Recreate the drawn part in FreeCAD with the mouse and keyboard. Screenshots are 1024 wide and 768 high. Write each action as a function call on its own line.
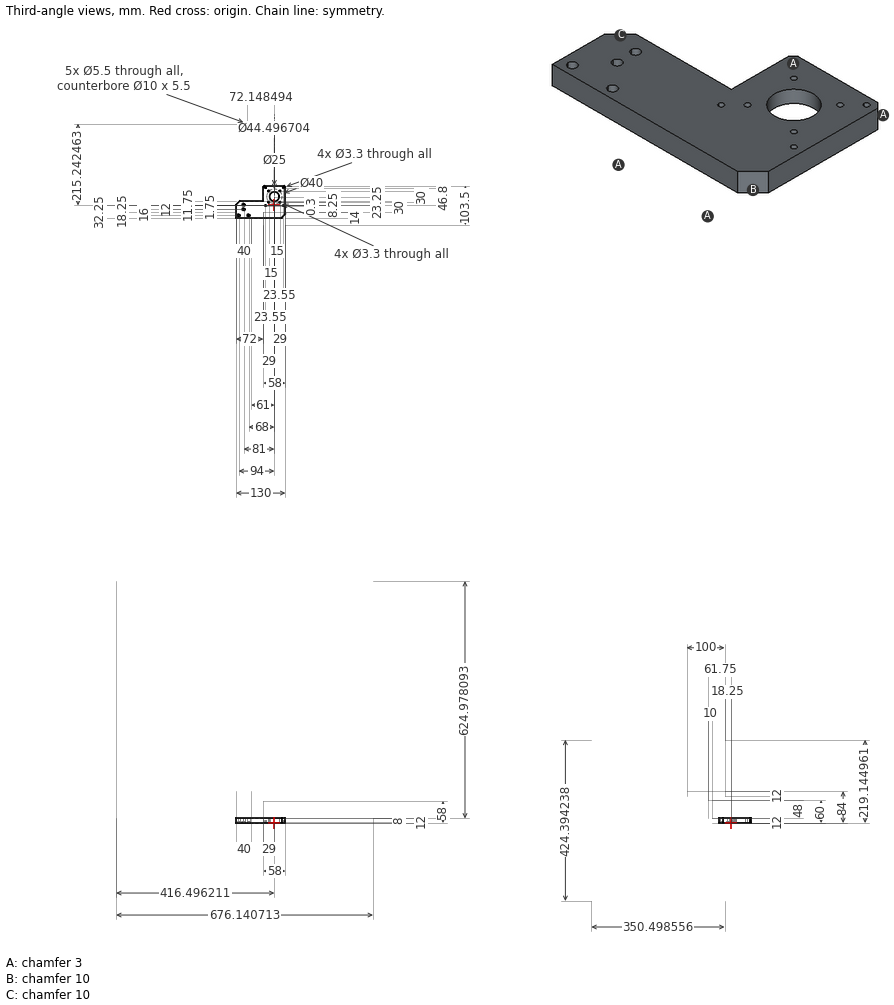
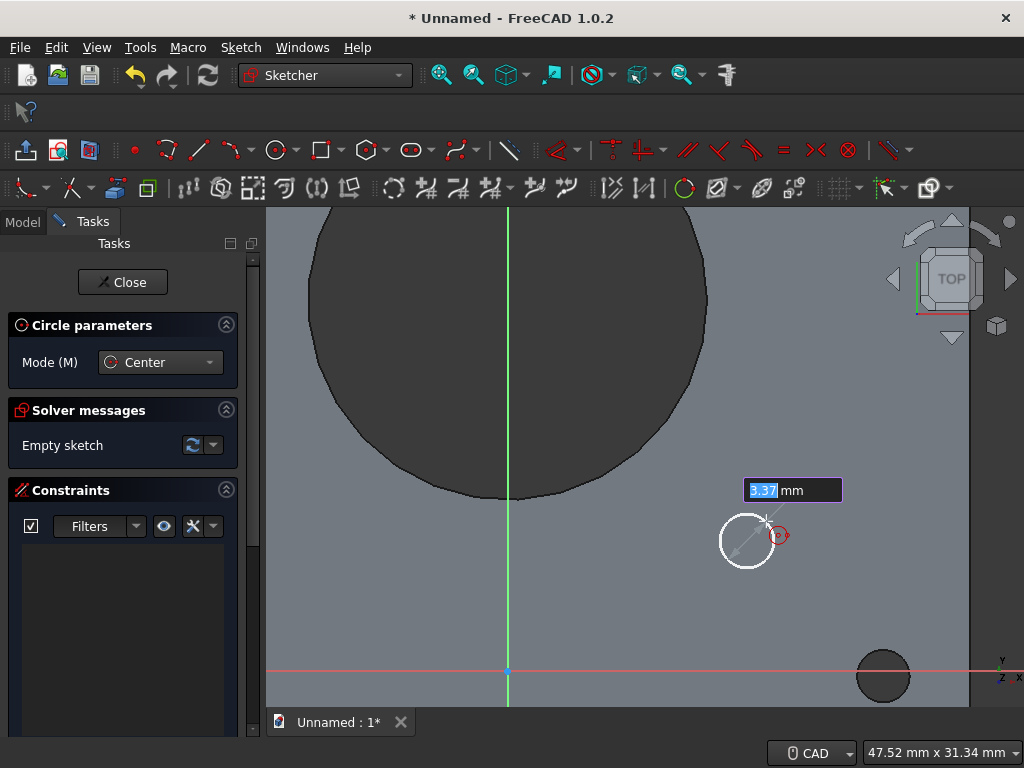
text(3.3)
key(Return)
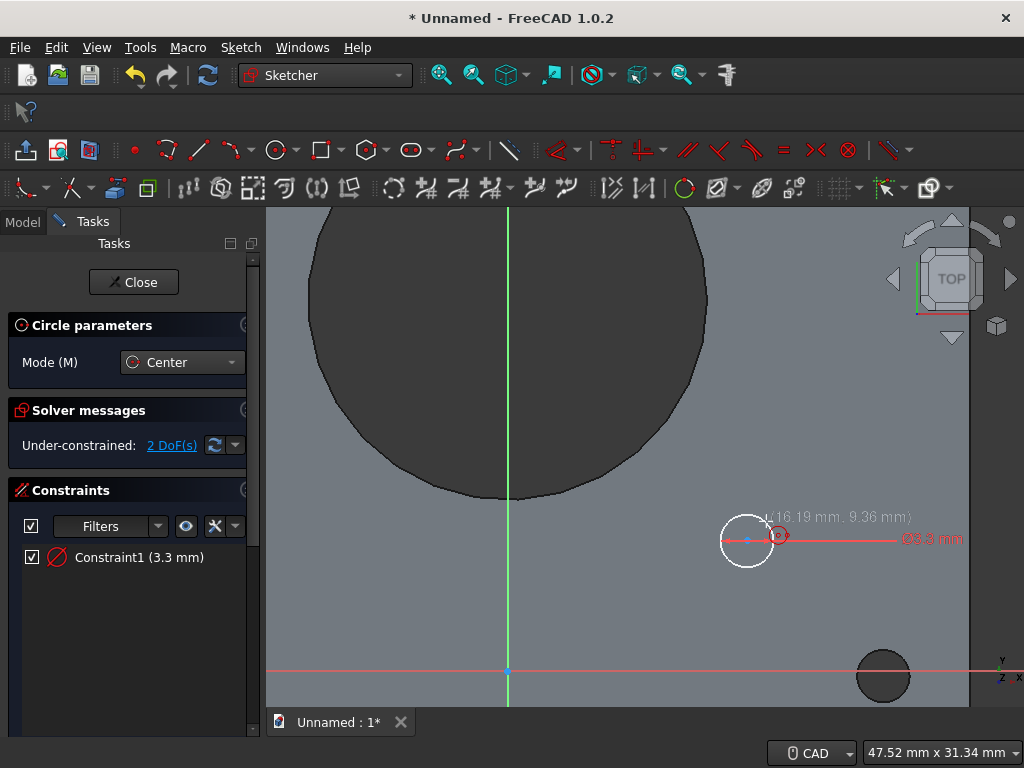
scroll(633, 542, down, 4)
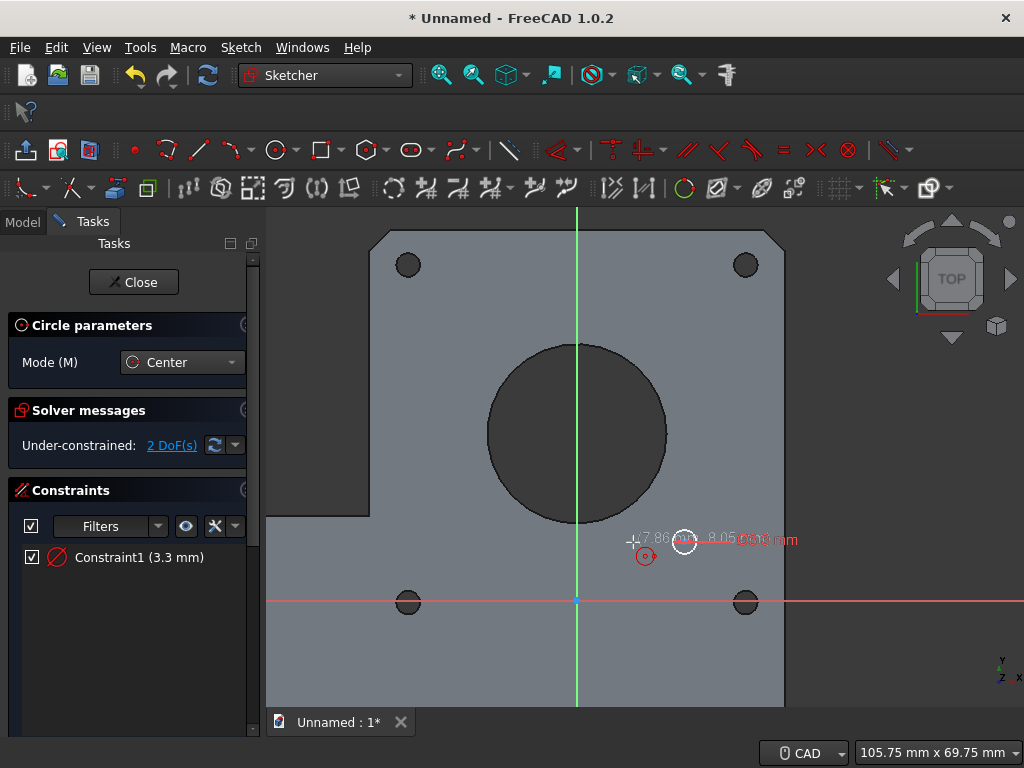
scroll(469, 541, up, 4)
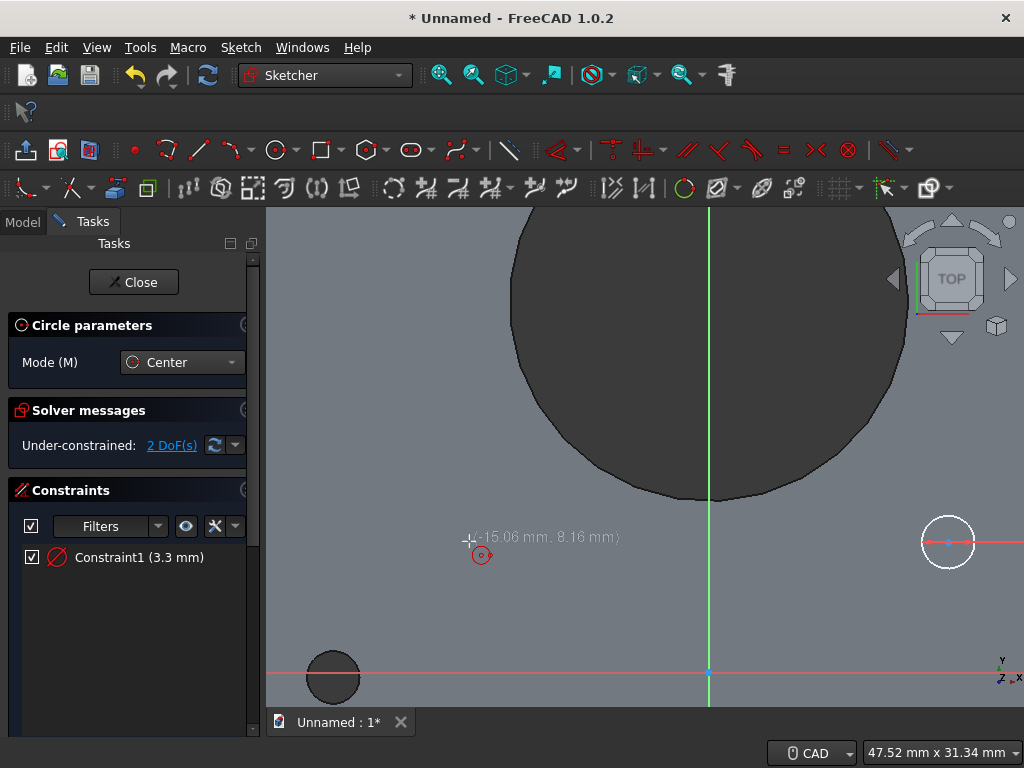
click(470, 541)
move(488, 522)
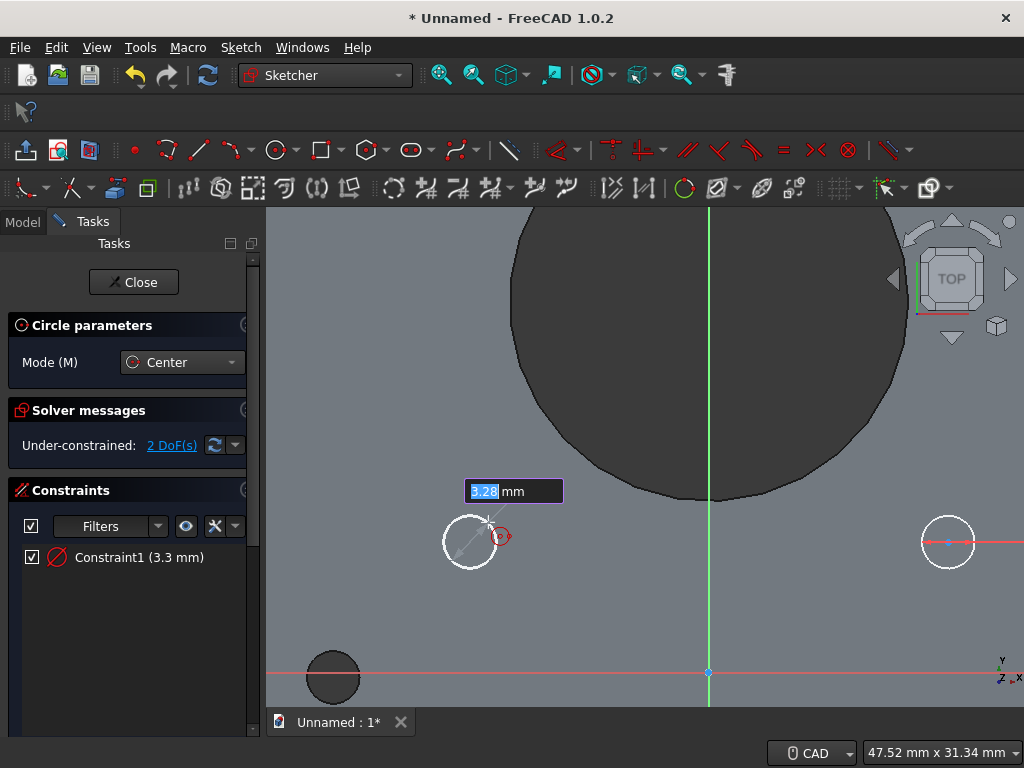
text(3.3)
key(Return)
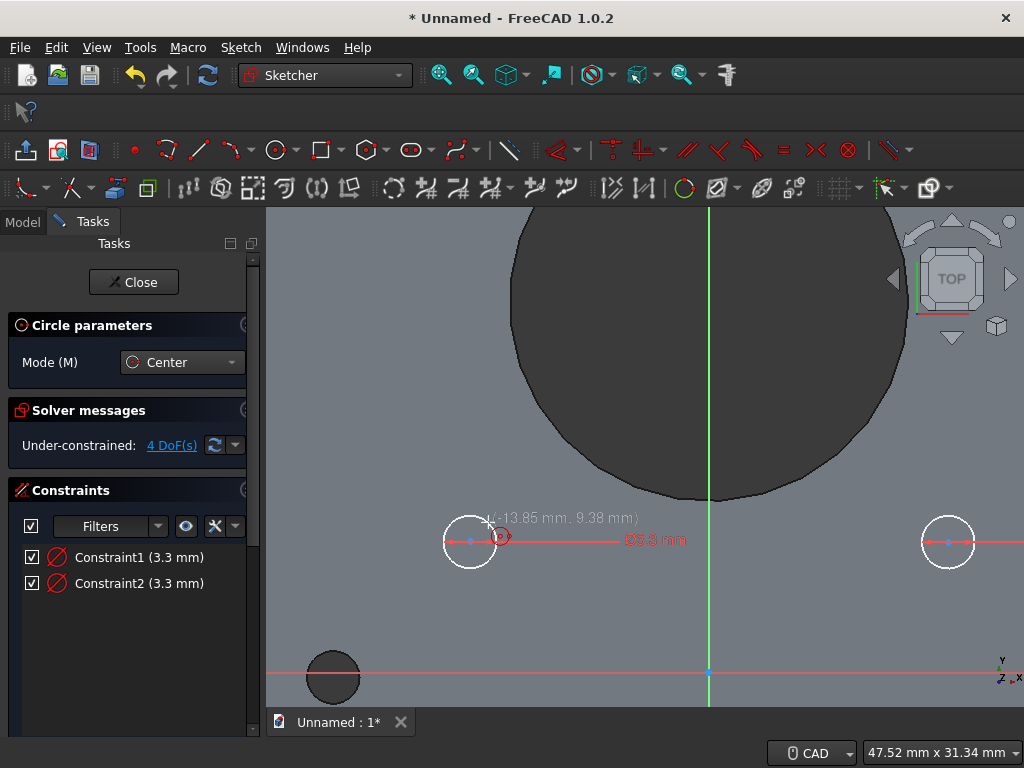
scroll(468, 541, down, 4)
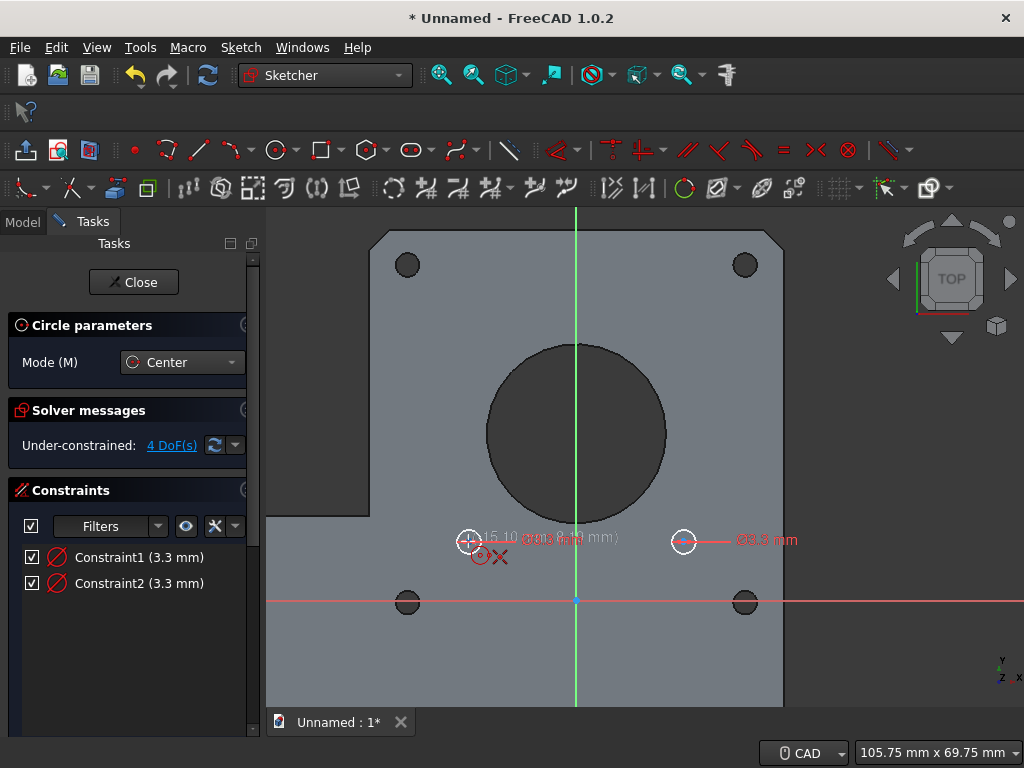
scroll(469, 326, up, 4)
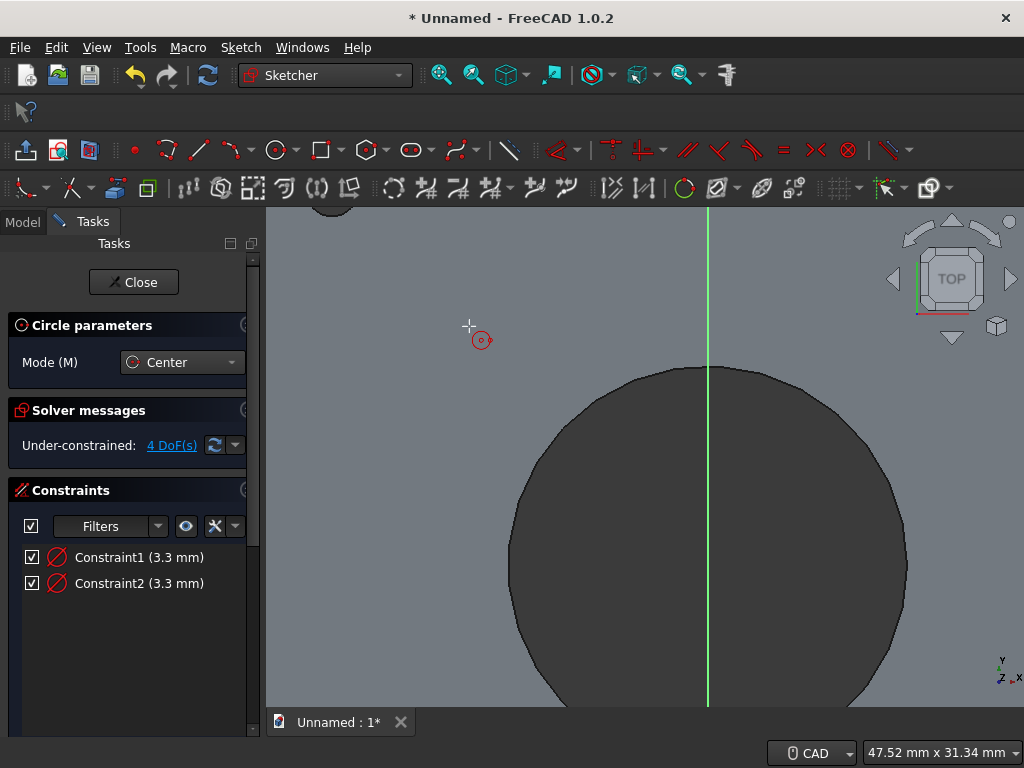
click(468, 326)
move(487, 308)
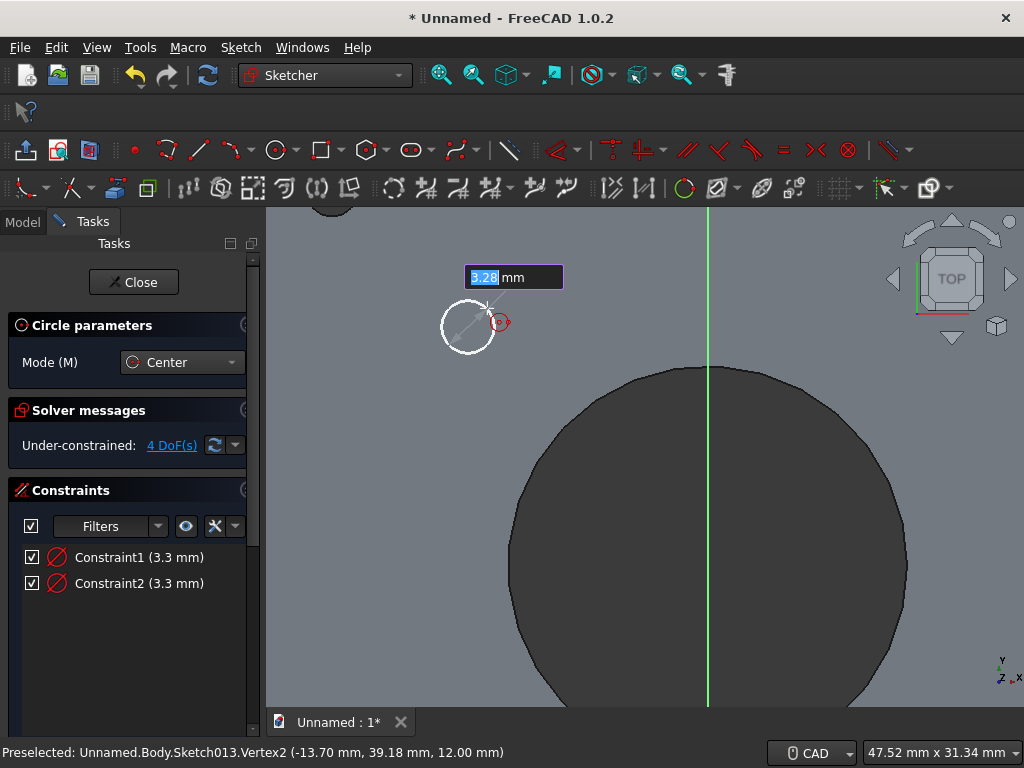
text(3.3)
key(Return)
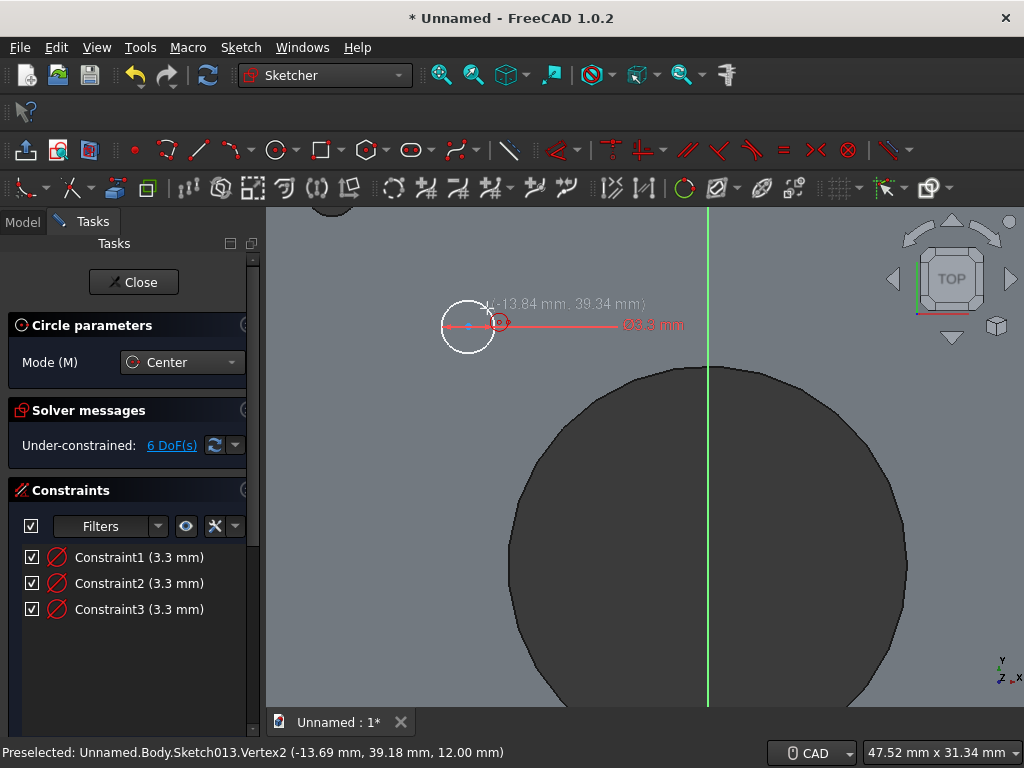
scroll(469, 325, down, 4)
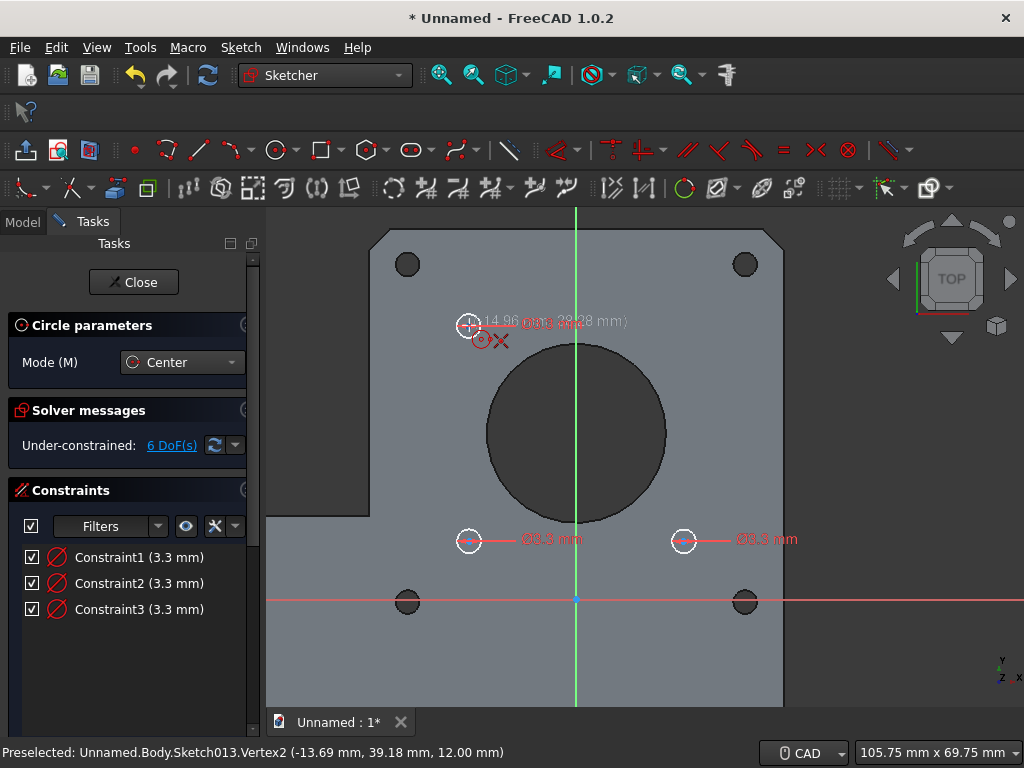
scroll(684, 326, up, 4)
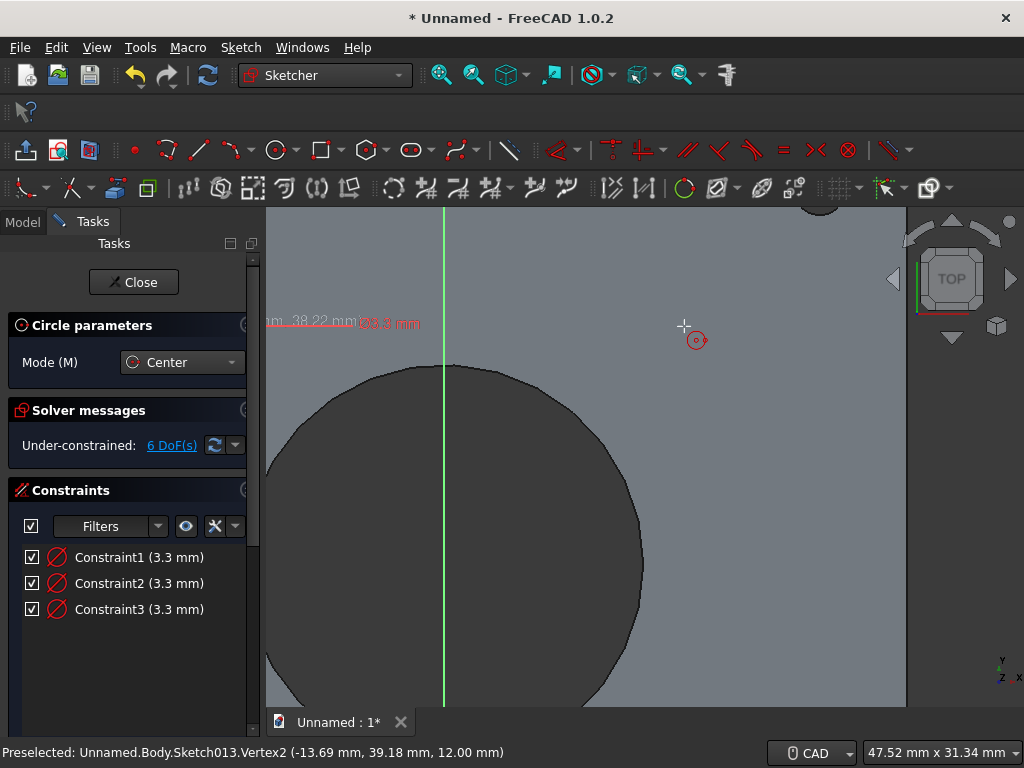
click(683, 325)
move(702, 307)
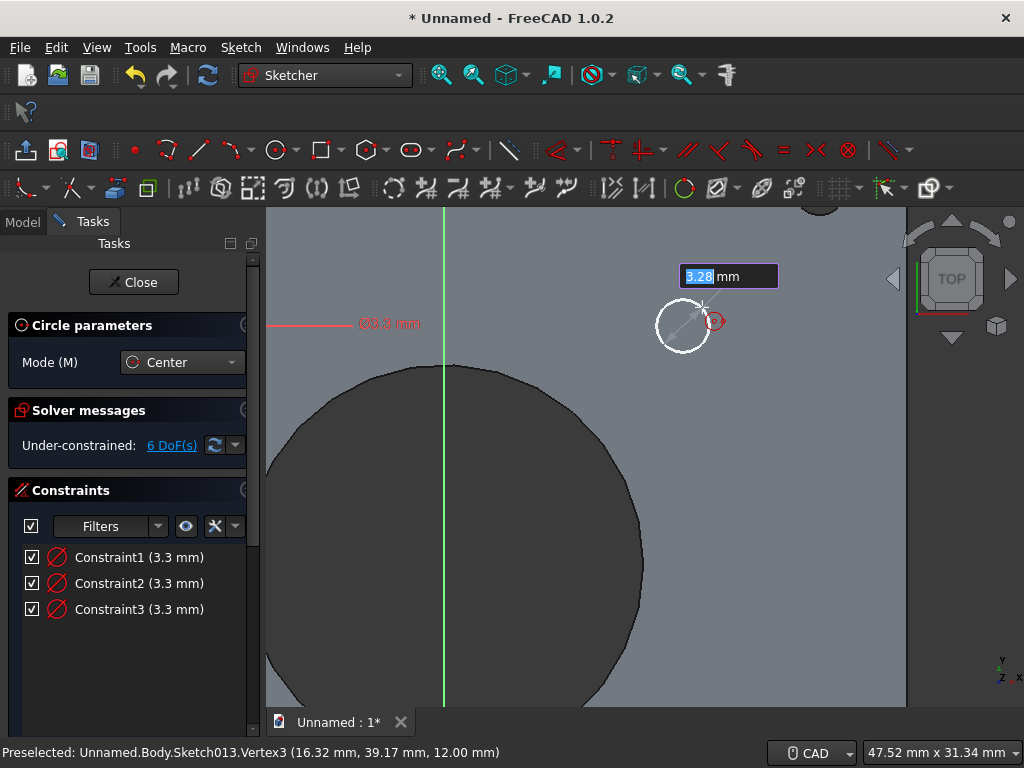
text(3.3)
key(Return)
key(Escape)